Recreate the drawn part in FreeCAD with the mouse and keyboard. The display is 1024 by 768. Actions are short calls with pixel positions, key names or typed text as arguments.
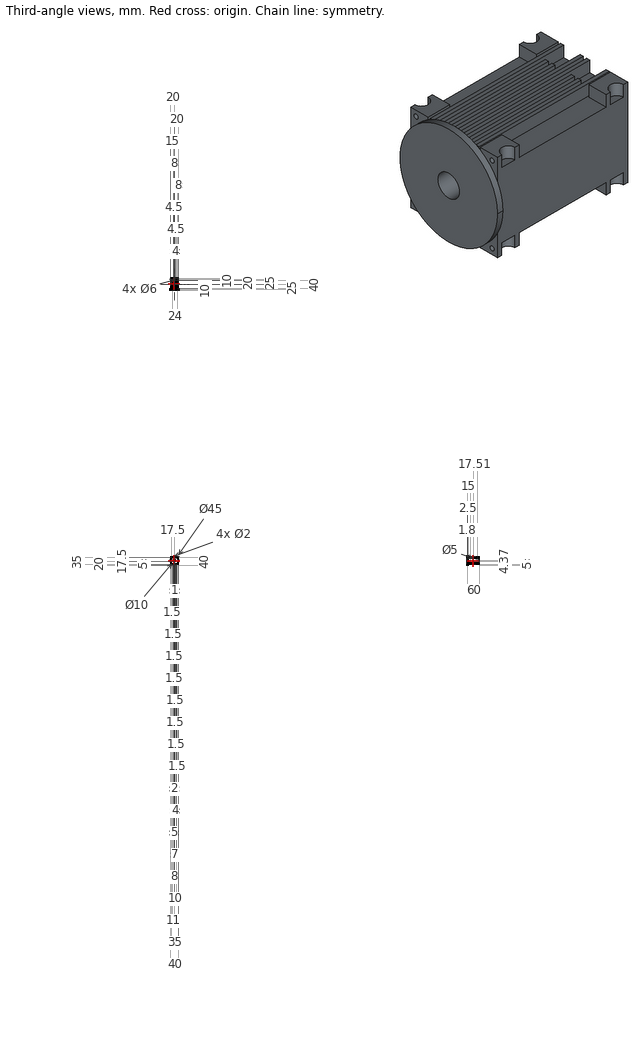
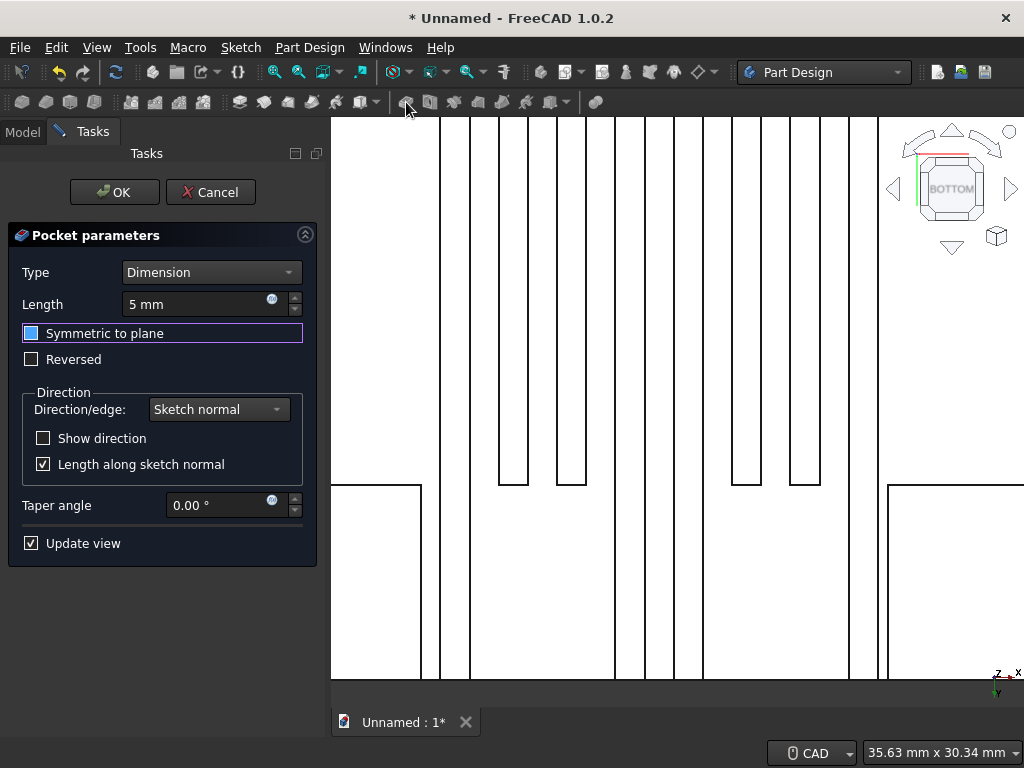
click(115, 192)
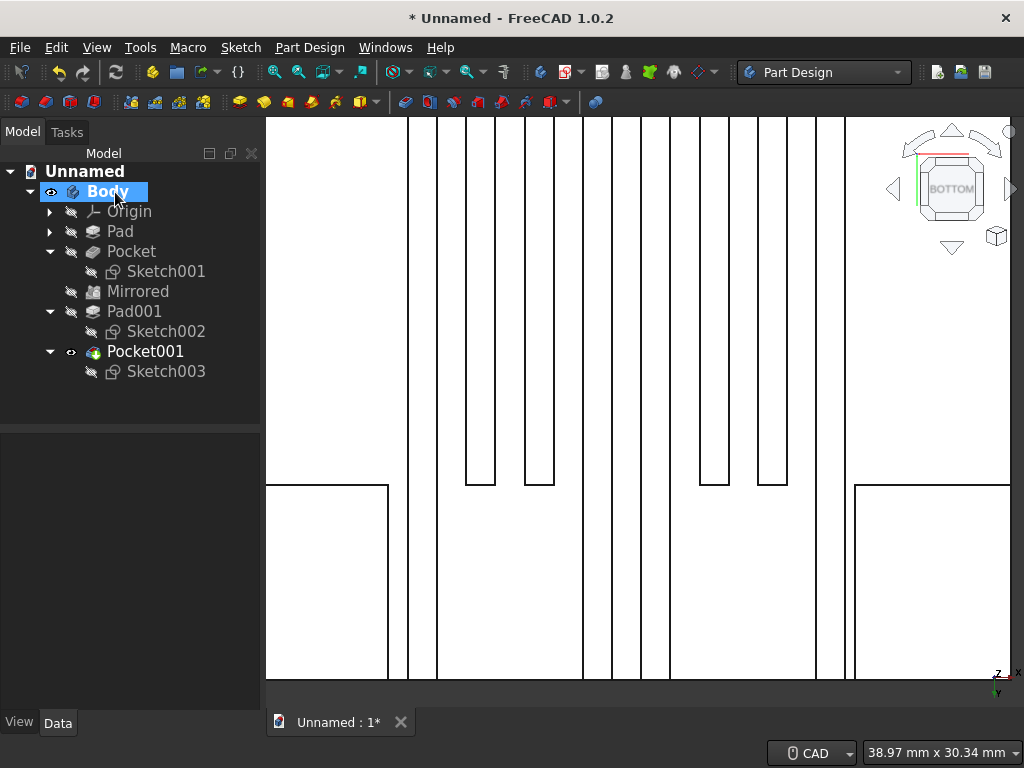
click(276, 72)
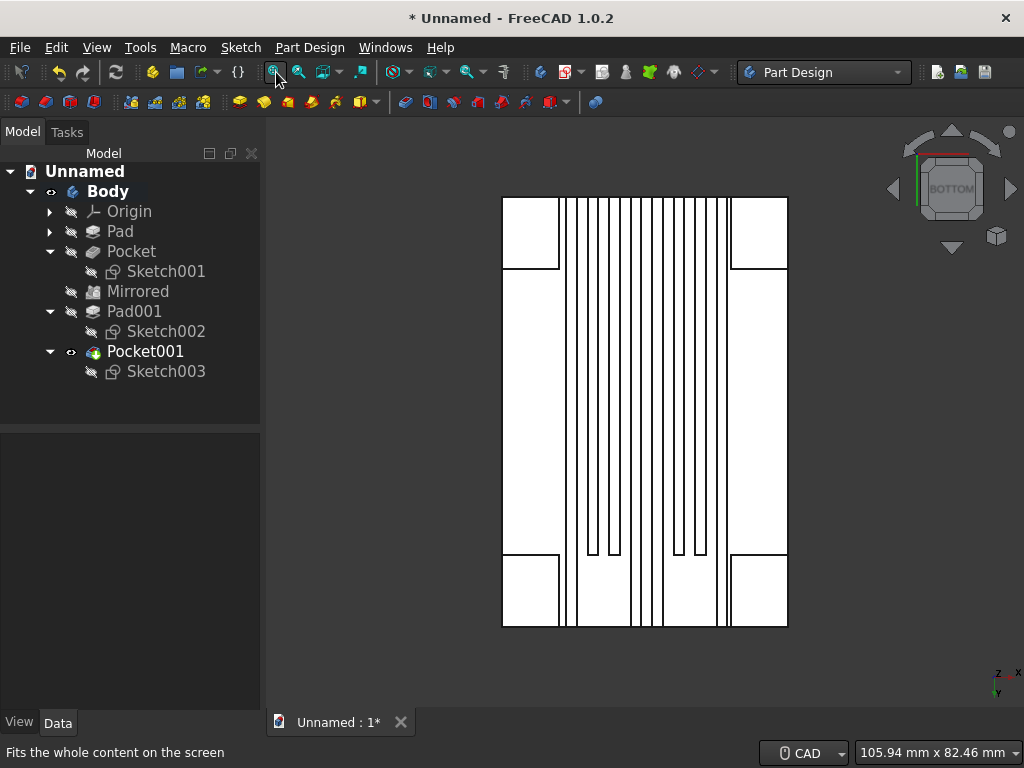
click(116, 312)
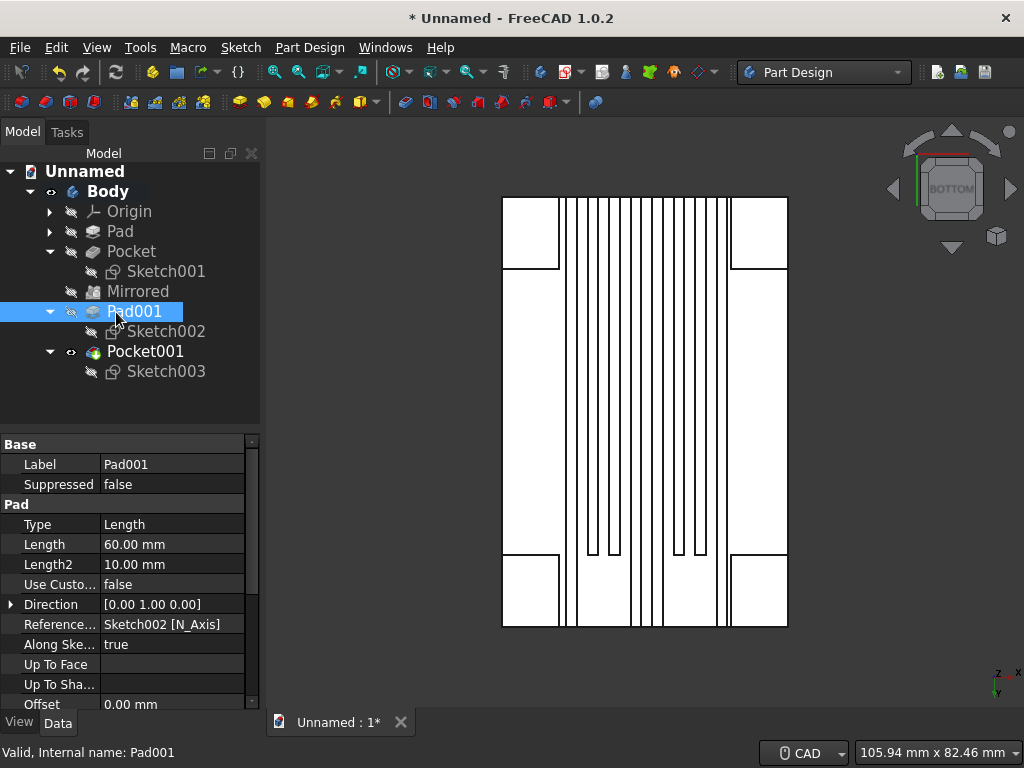
click(116, 352, ctrl)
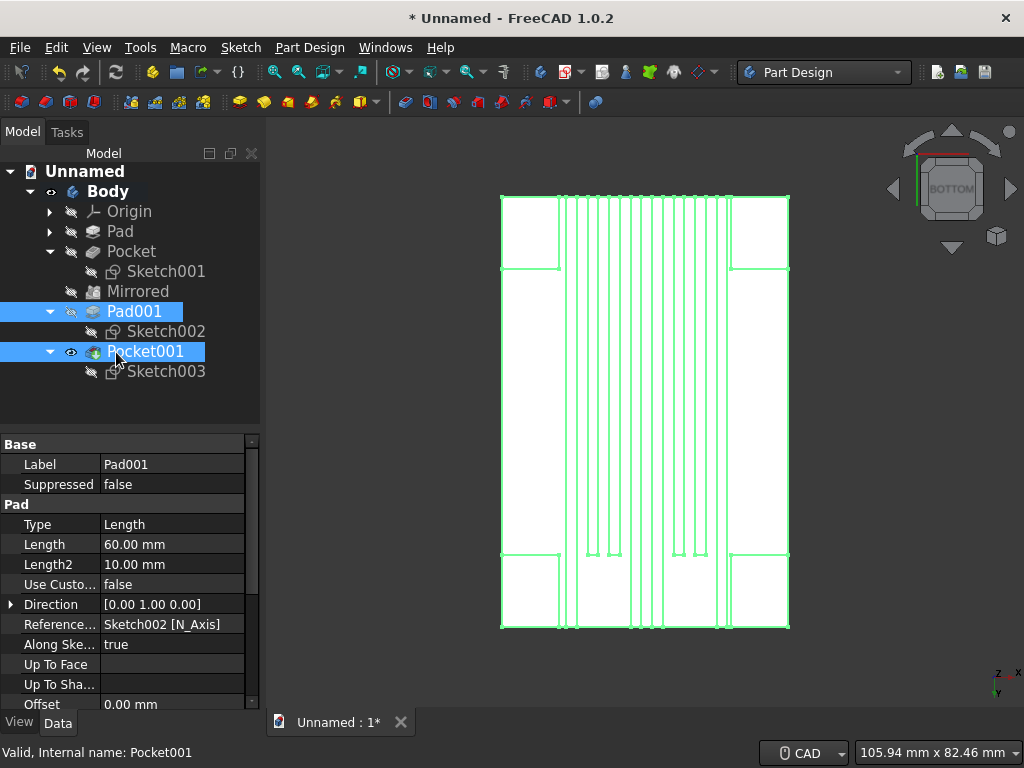
click(132, 102)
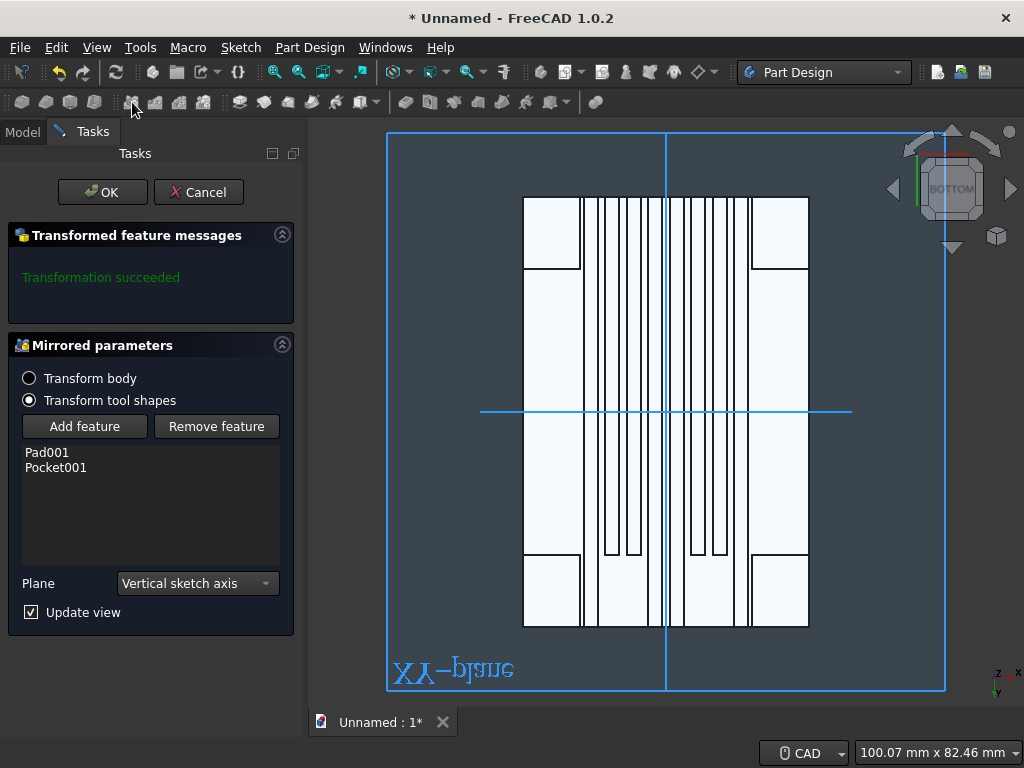
click(198, 584)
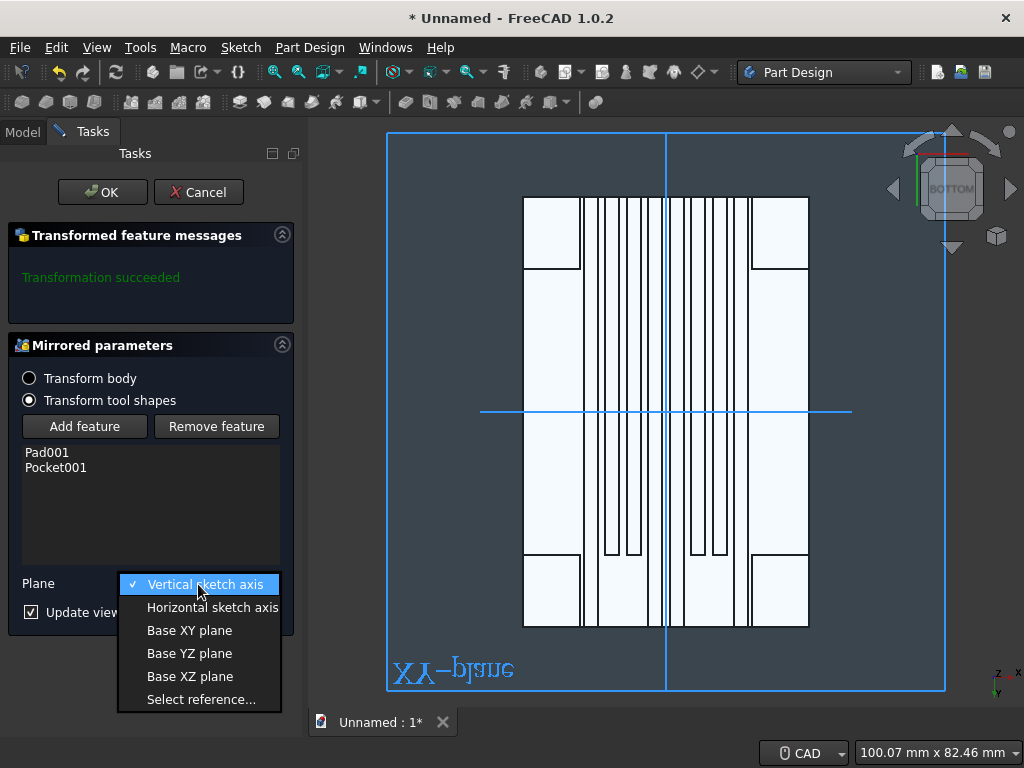
click(198, 630)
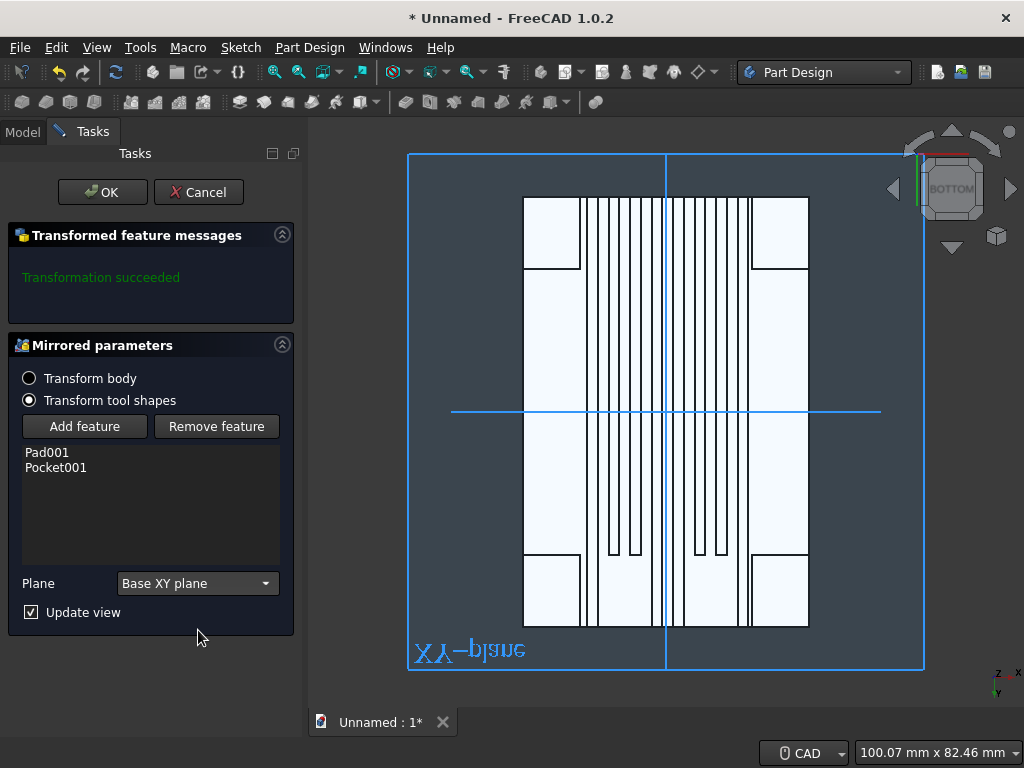
click(103, 192)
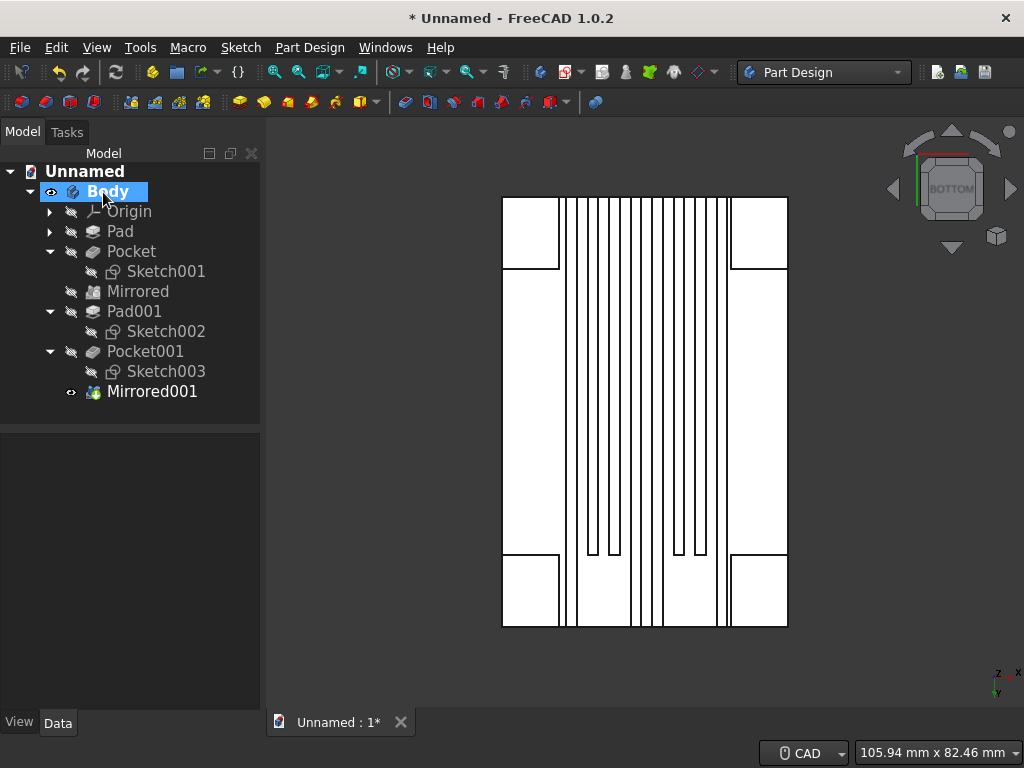
scroll(722, 595, up, 5)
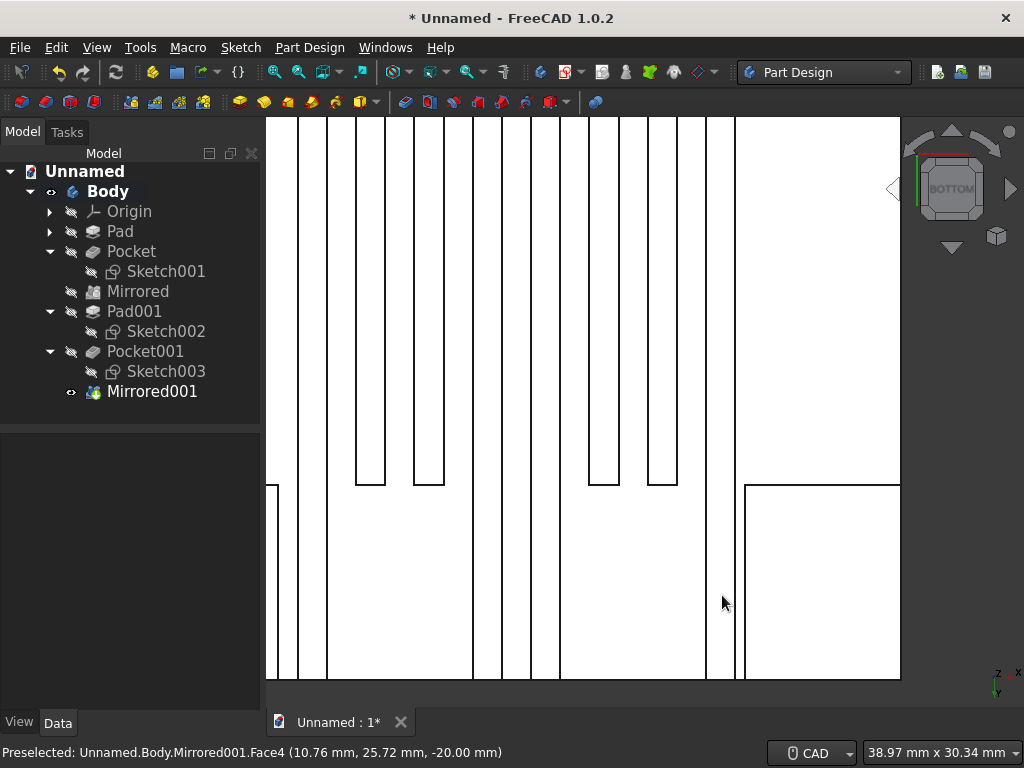
click(721, 595)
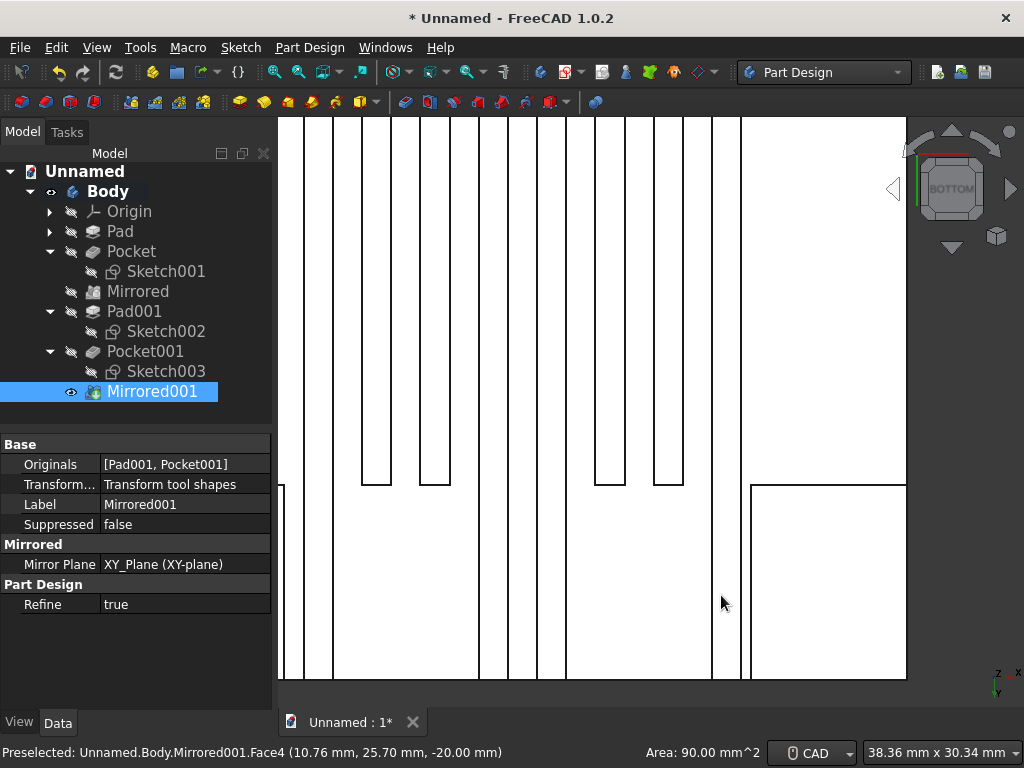
click(566, 72)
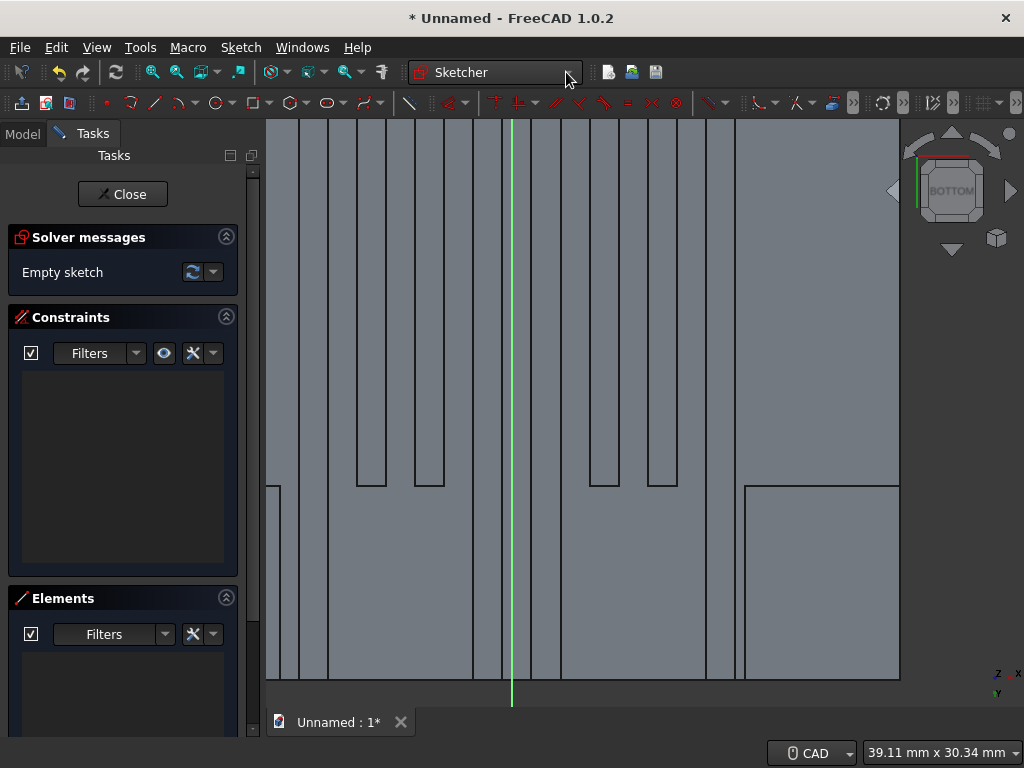
scroll(614, 596, down, 5)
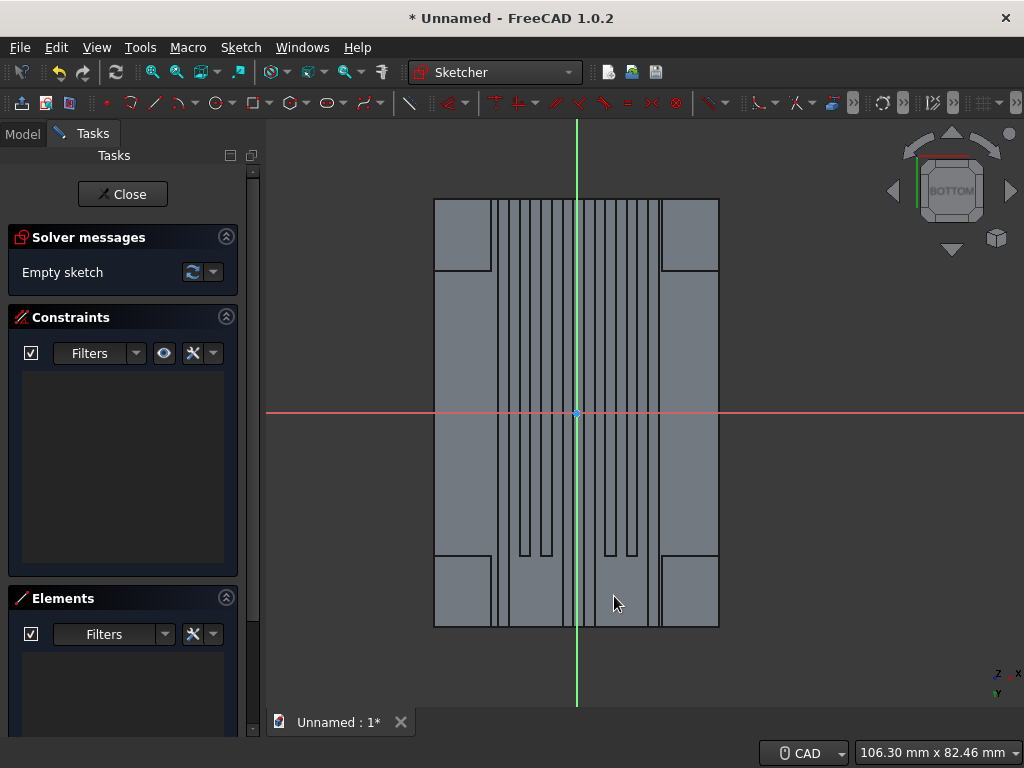
click(216, 104)